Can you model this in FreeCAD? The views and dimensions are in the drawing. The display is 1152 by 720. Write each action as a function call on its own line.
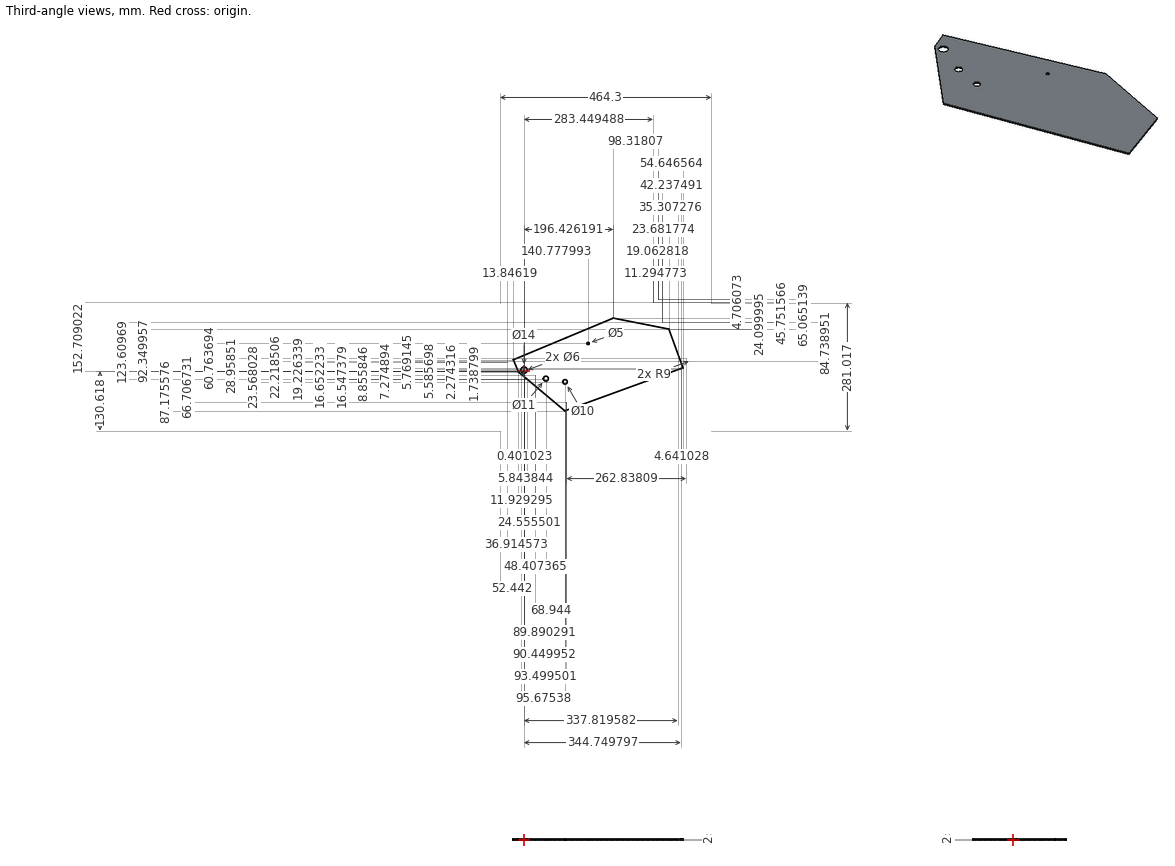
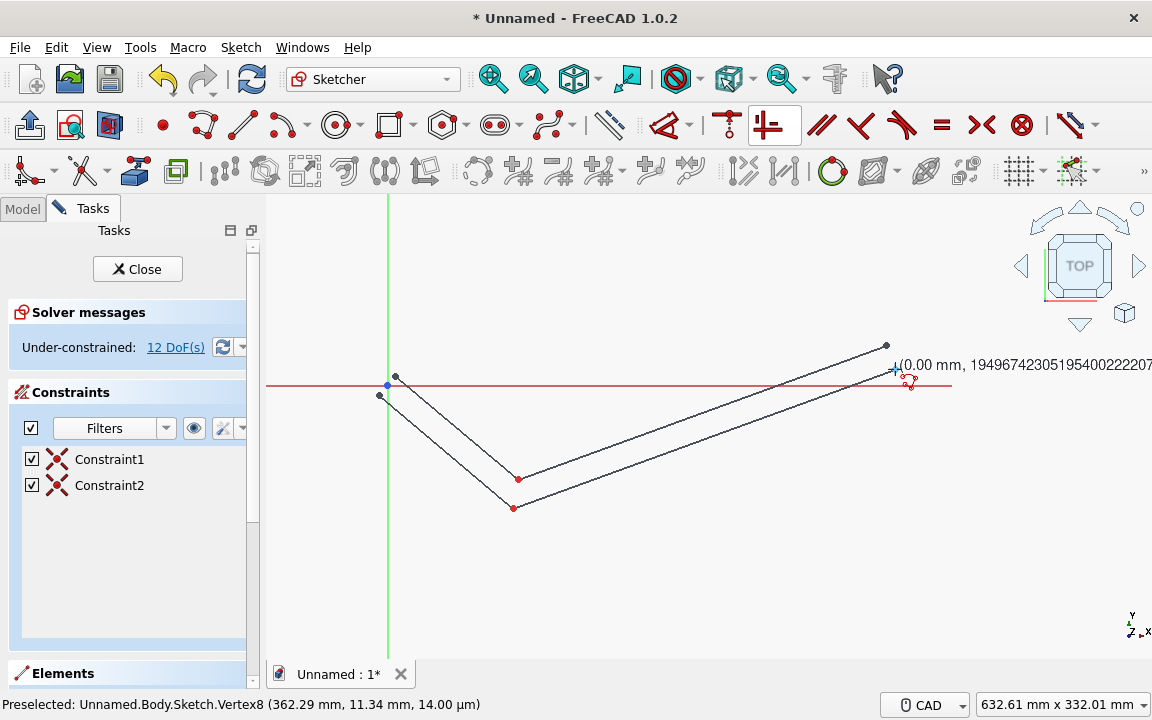
click(310, 126)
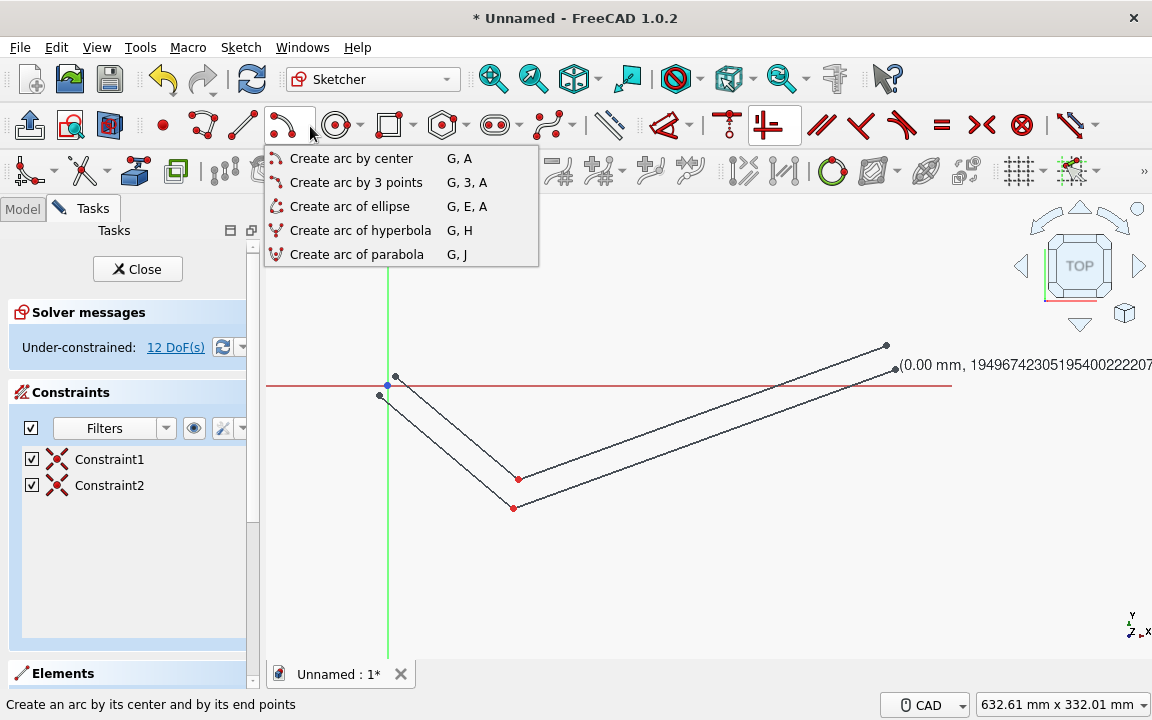
click(402, 182)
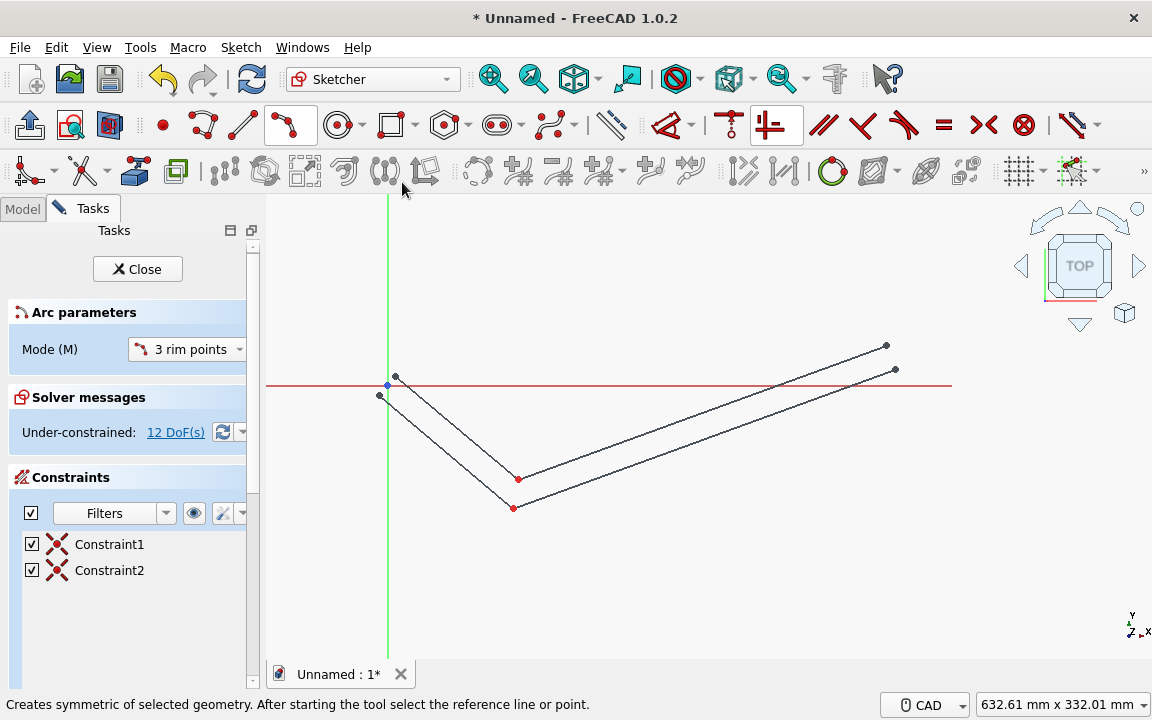
scroll(396, 376, up, 4)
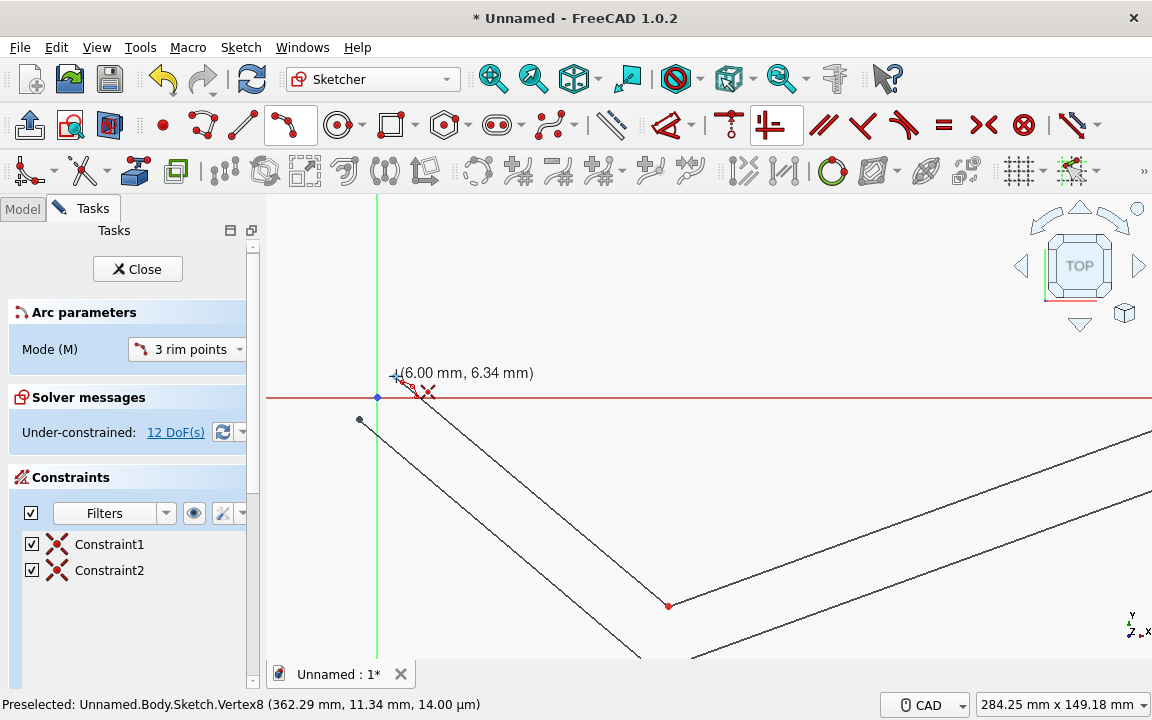
click(395, 377)
click(359, 420)
click(356, 379)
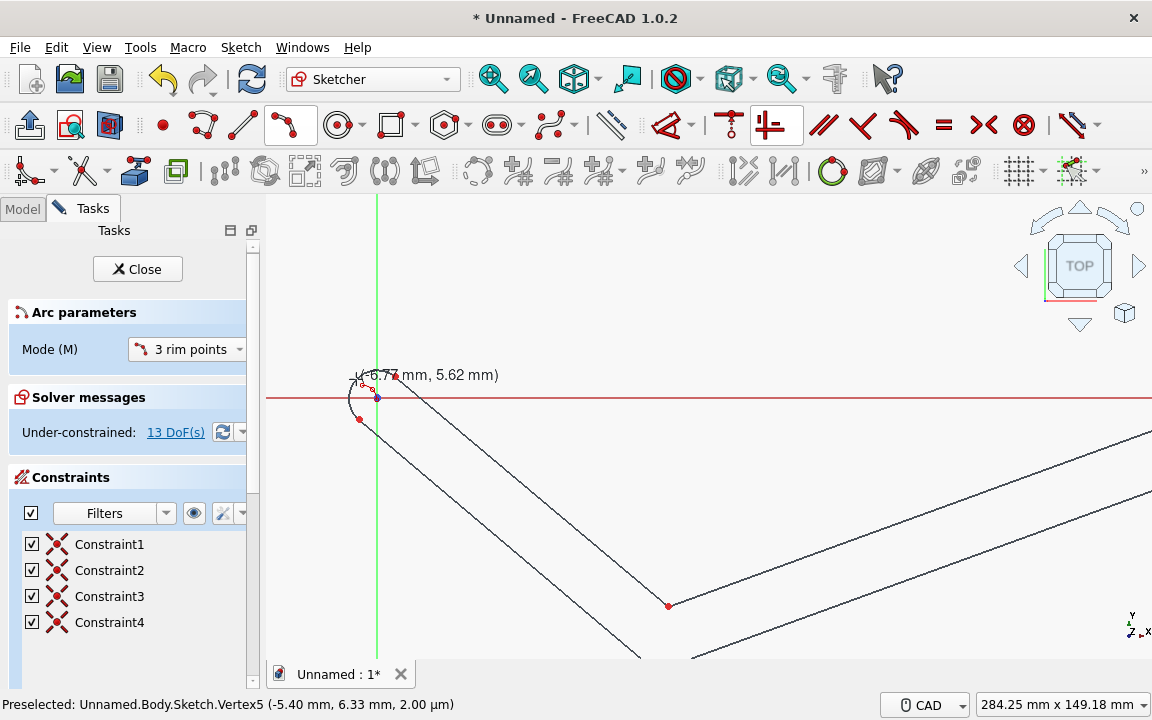
scroll(396, 376, down, 4)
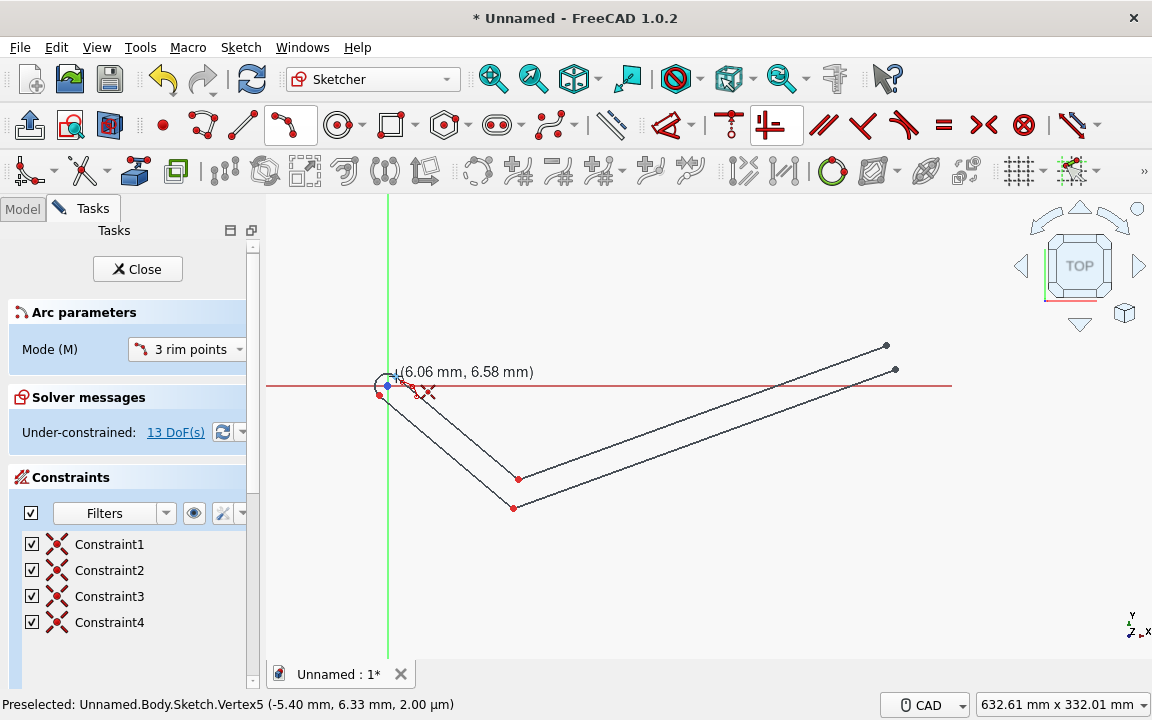
click(895, 370)
click(887, 346)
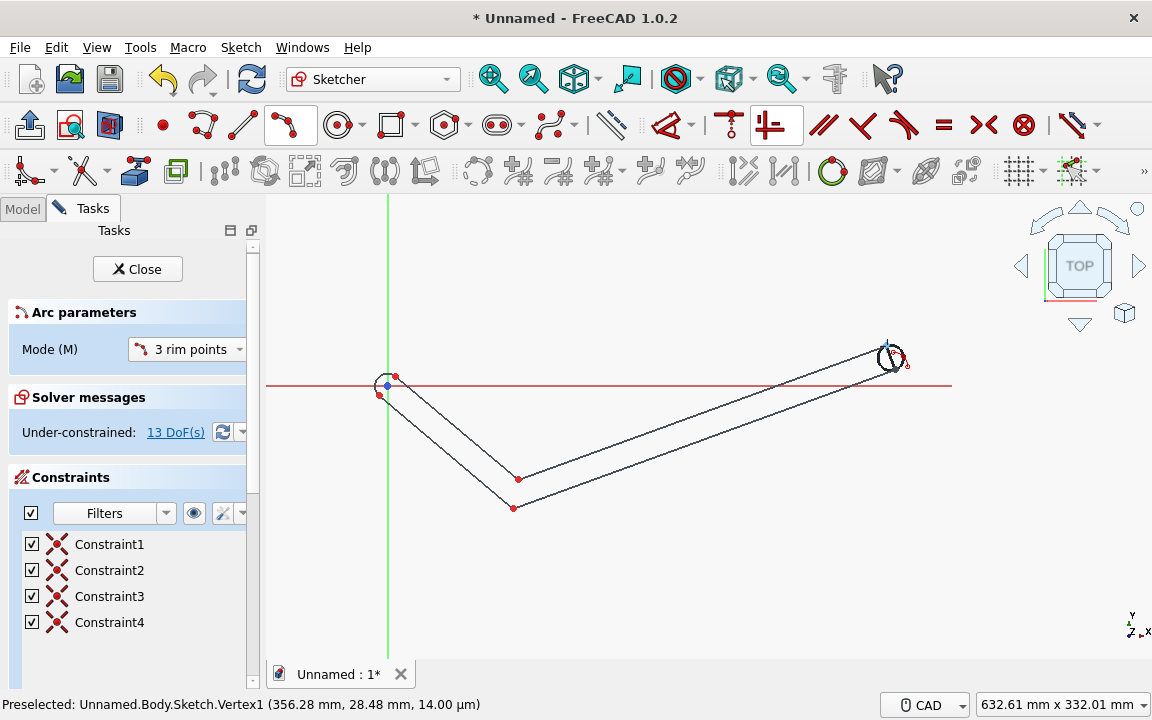
scroll(903, 353, up, 2)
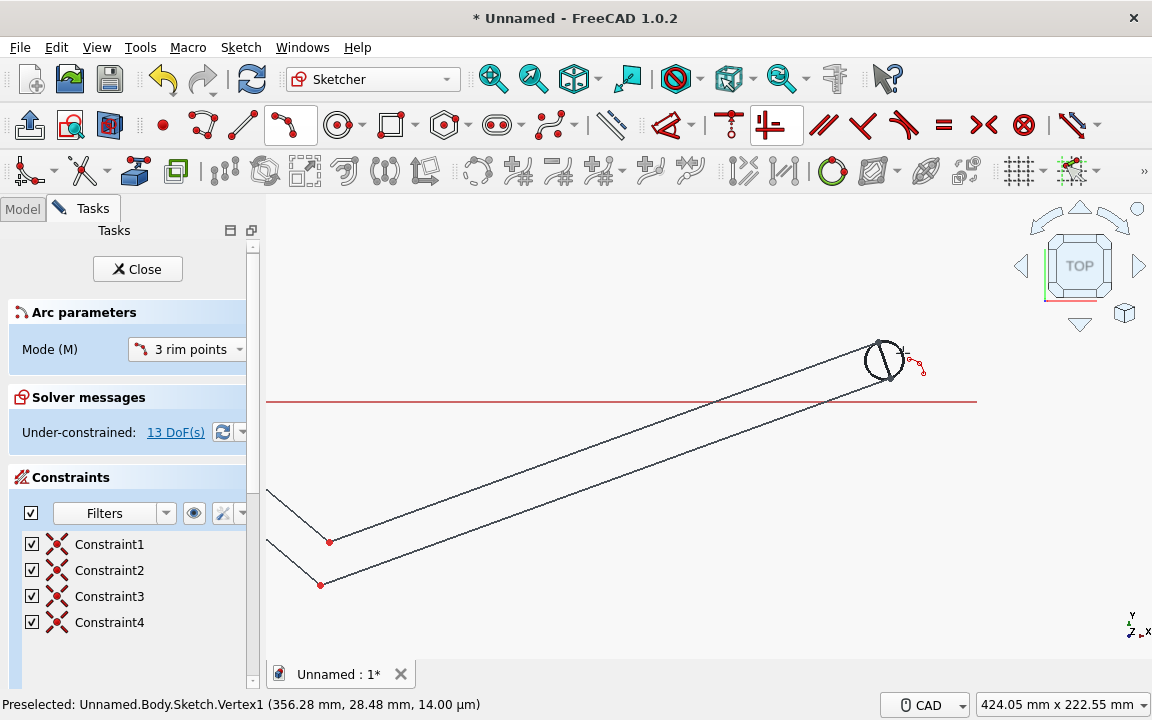
click(902, 353)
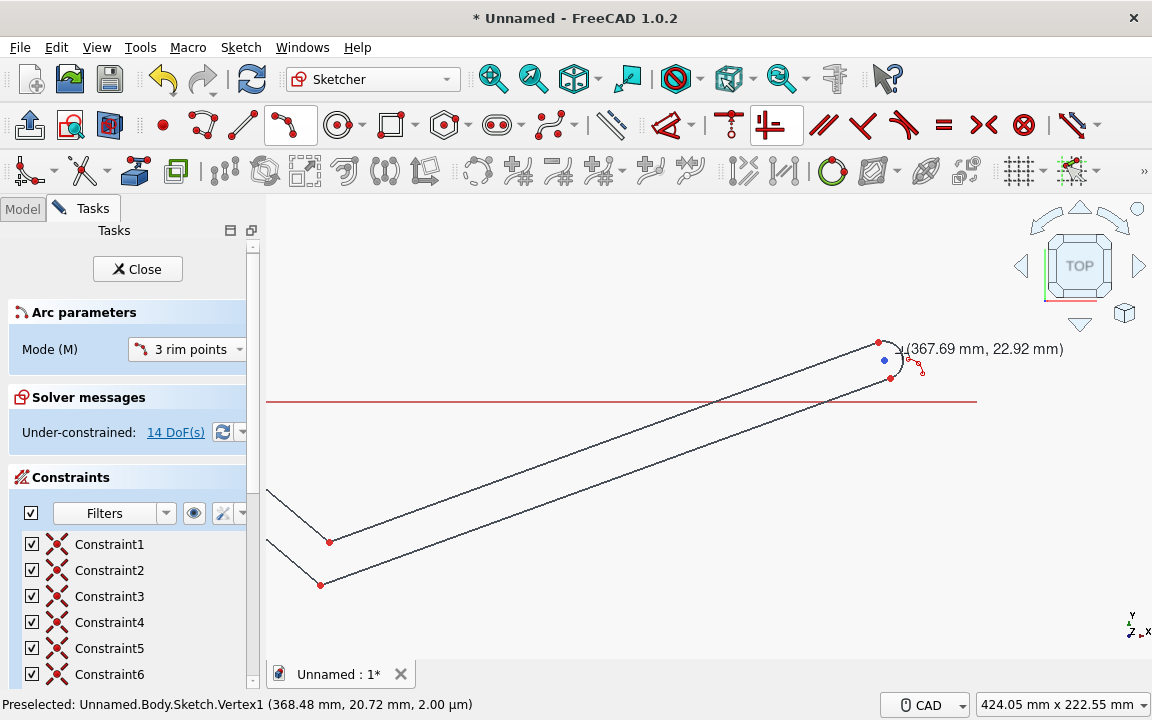
key(g)
key(c)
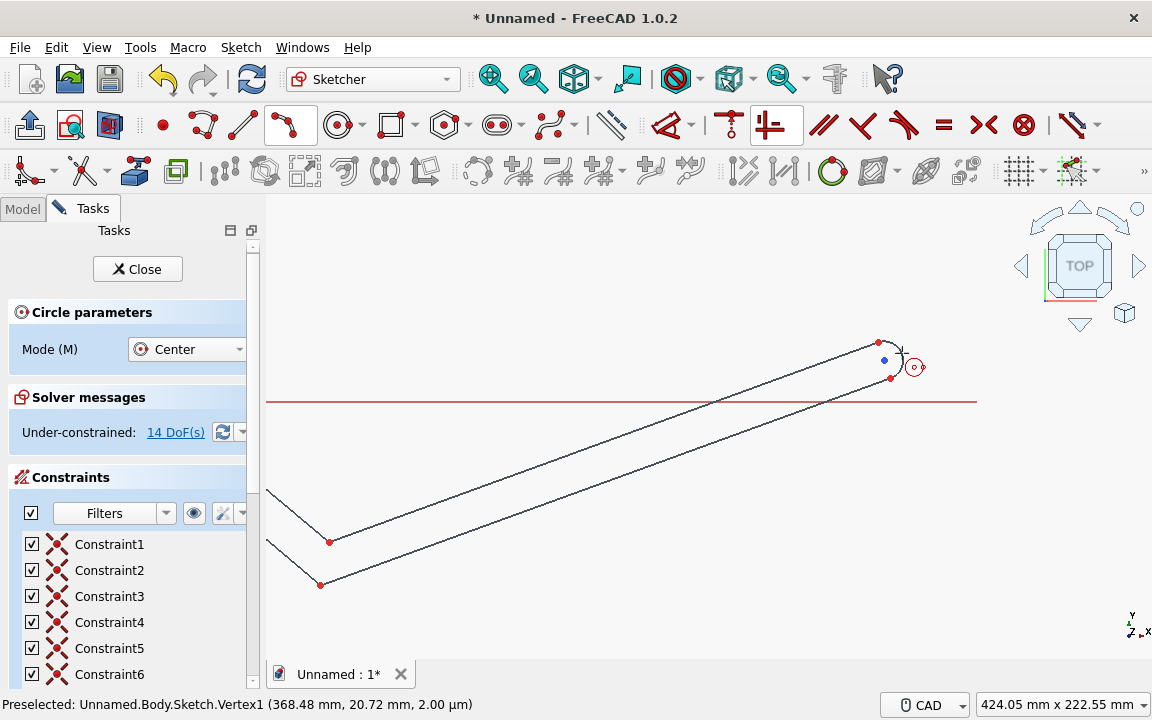
scroll(904, 353, down, 2)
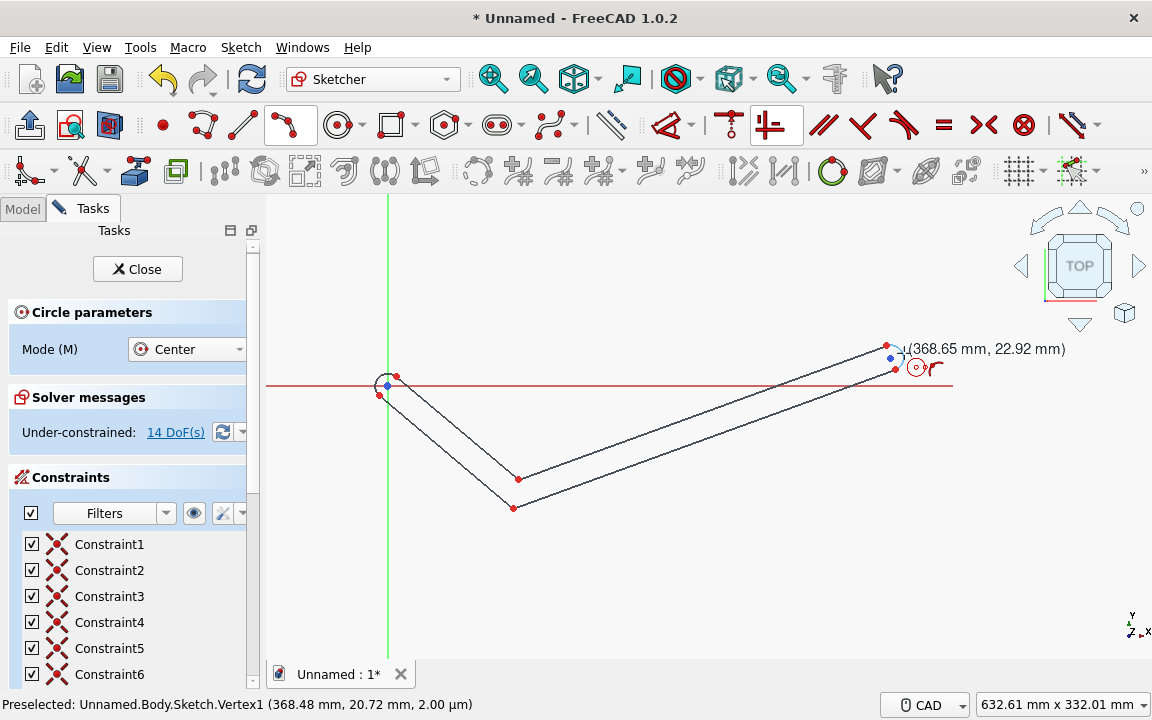
scroll(388, 386, up, 9)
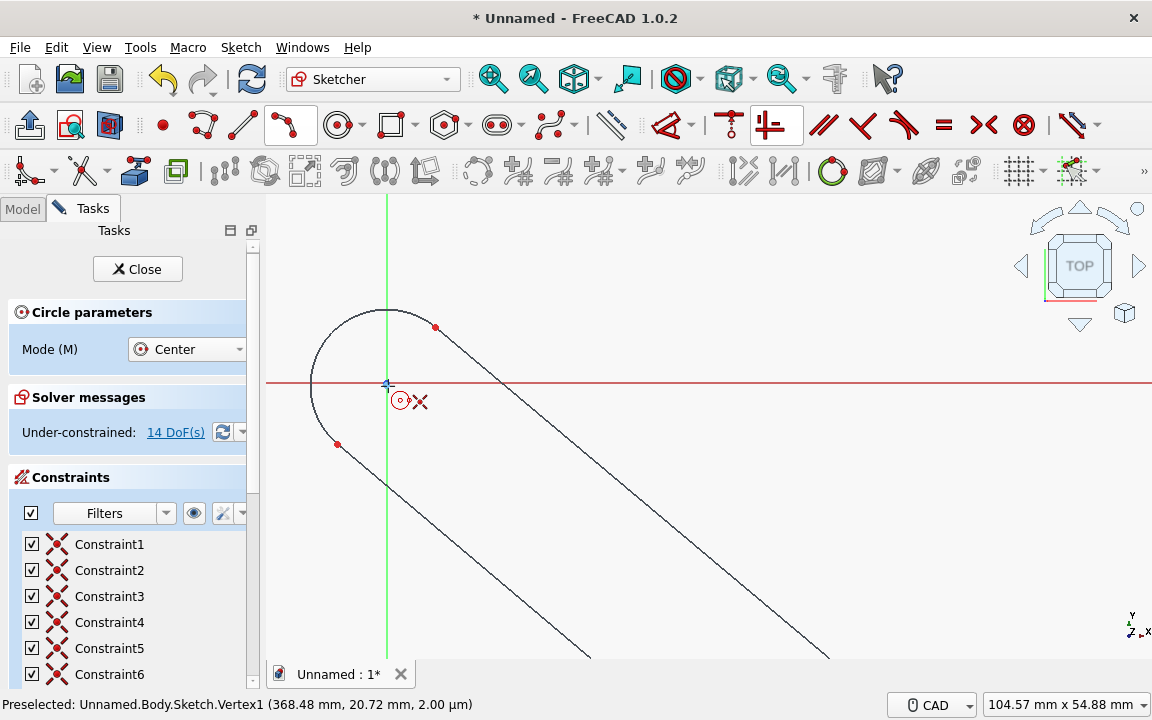
scroll(388, 386, down, 9)